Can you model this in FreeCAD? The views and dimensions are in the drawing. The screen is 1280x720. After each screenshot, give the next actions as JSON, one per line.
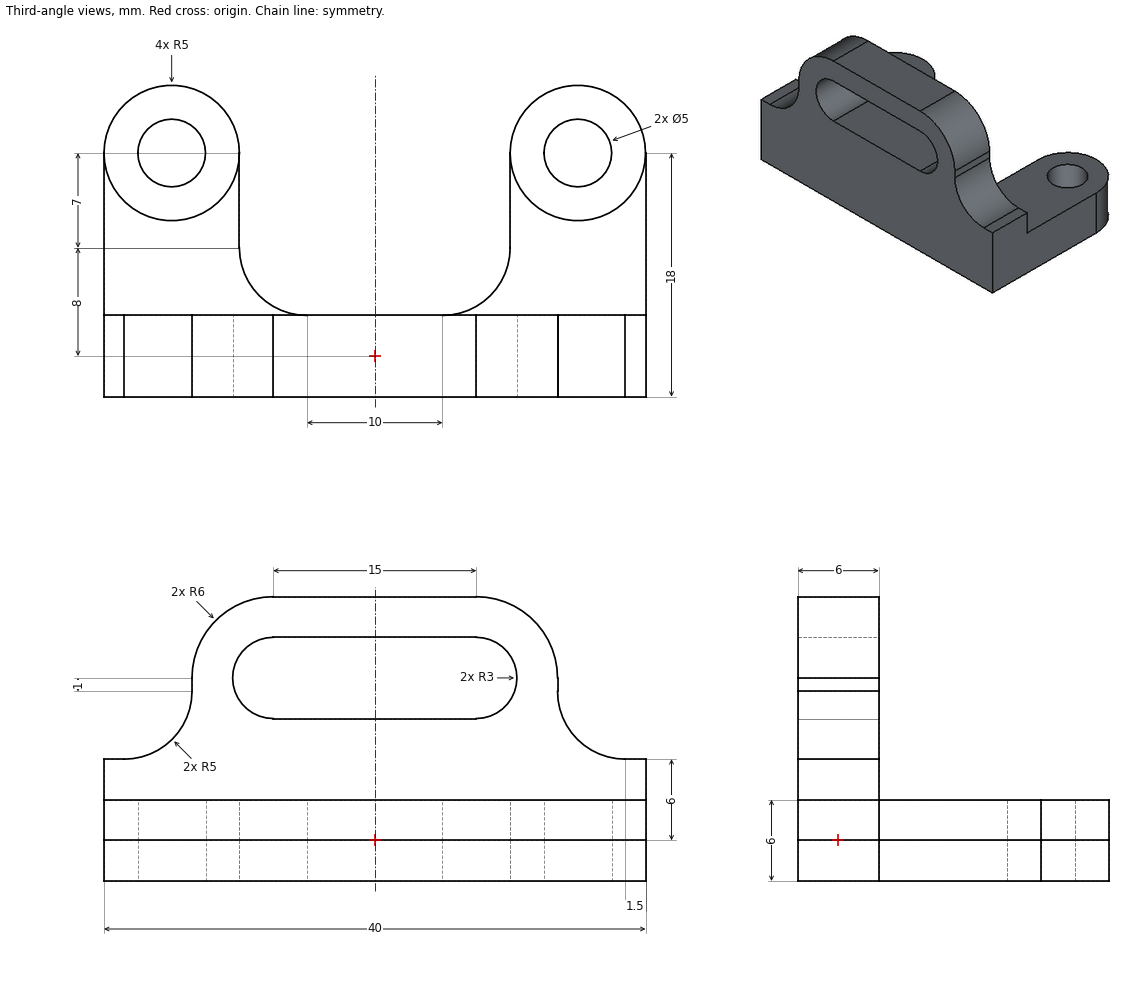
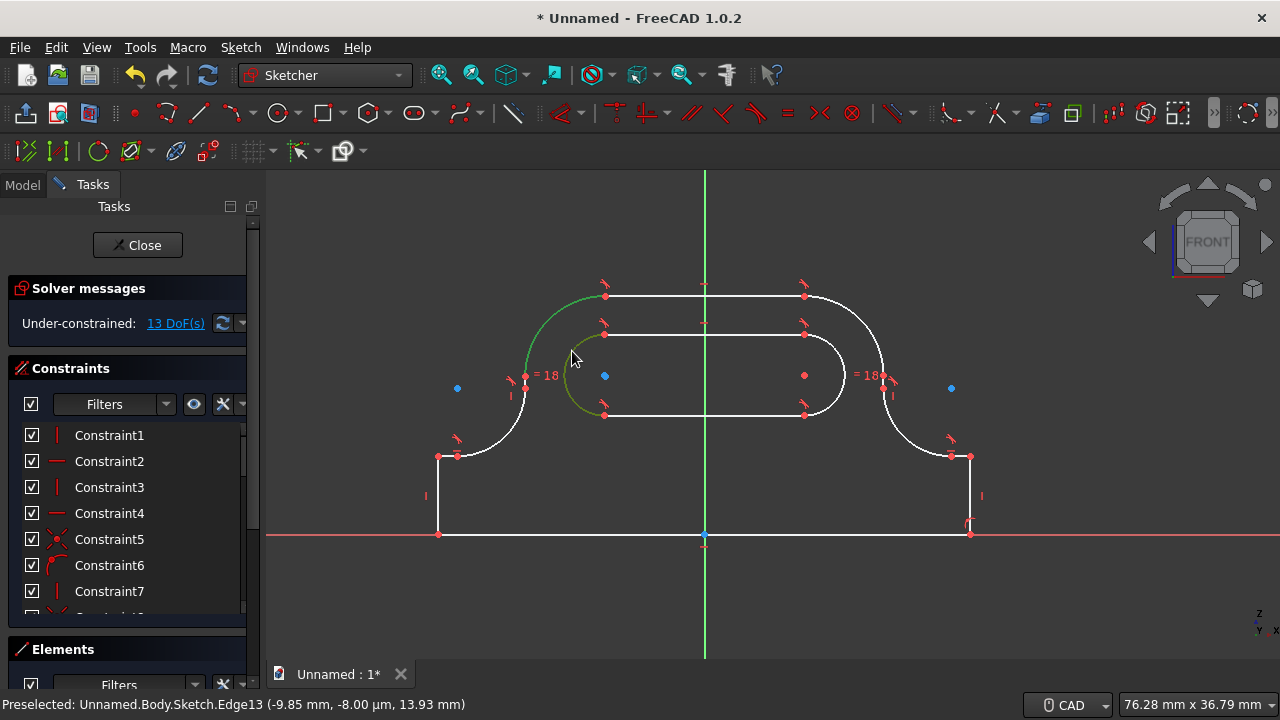
{"action": "left_click", "coordinate": [616, 114]}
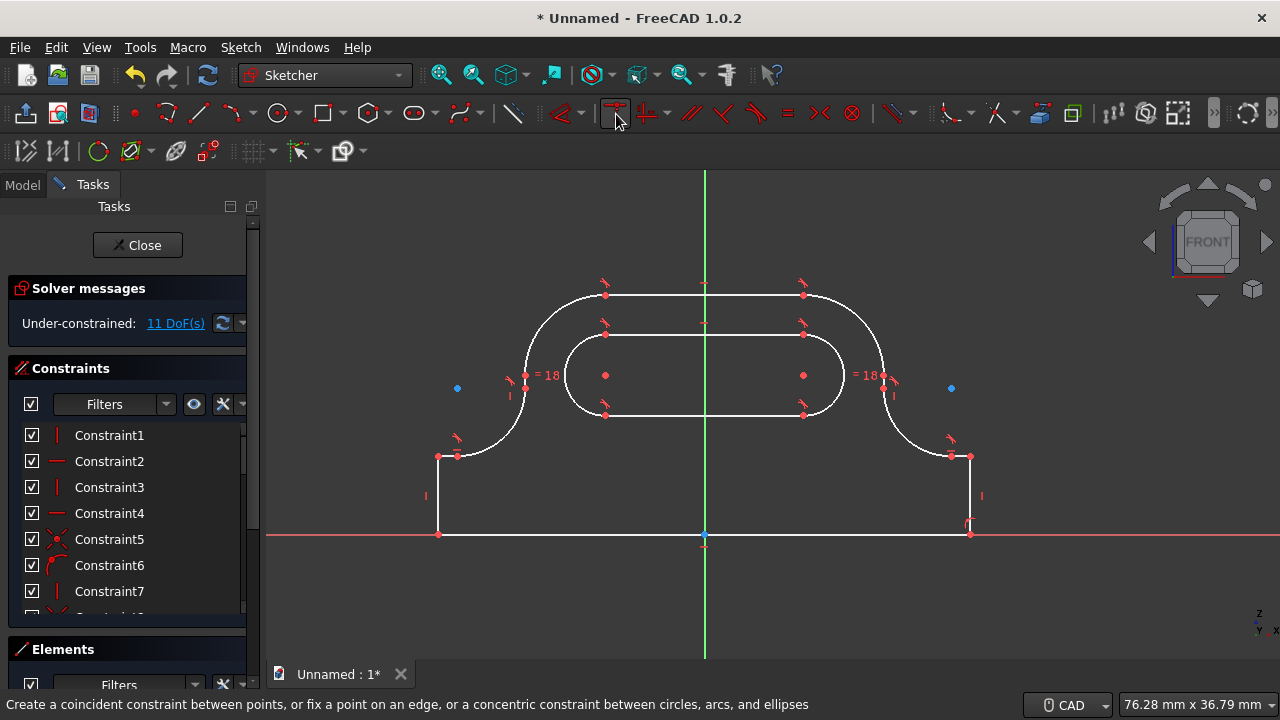
{"action": "left_click", "coordinate": [891, 419]}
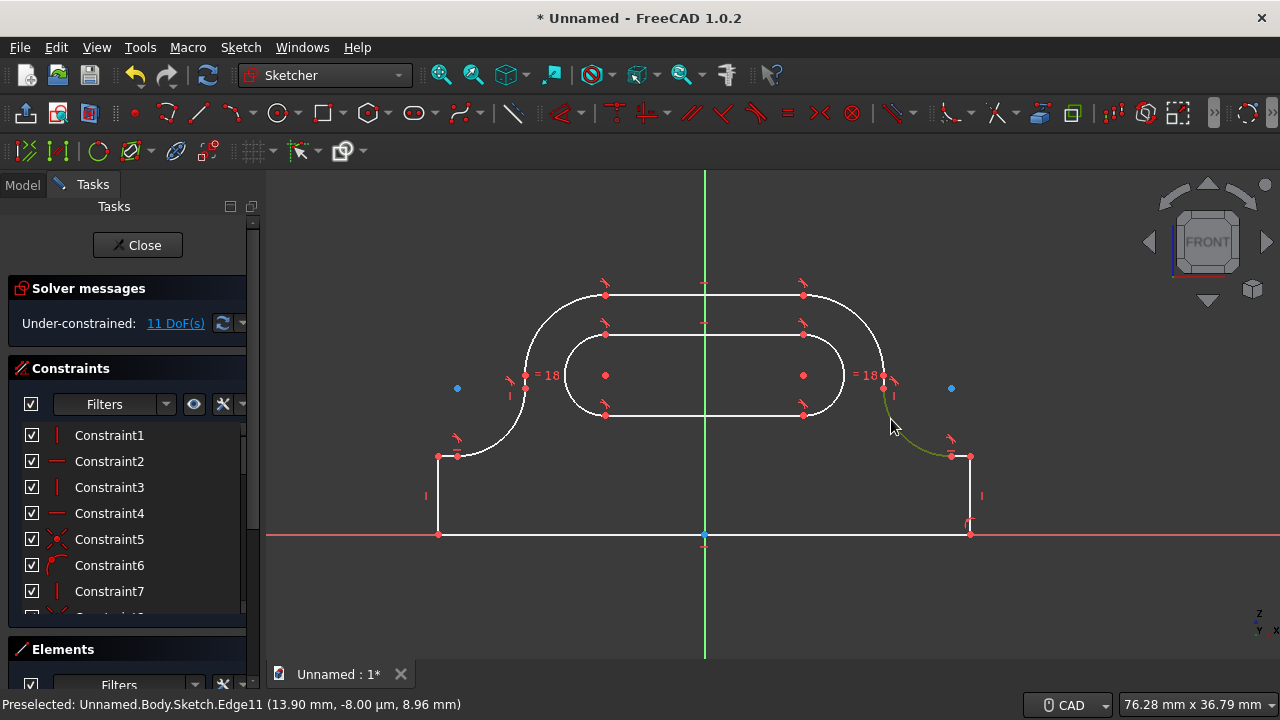
{"action": "left_click", "coordinate": [488, 449]}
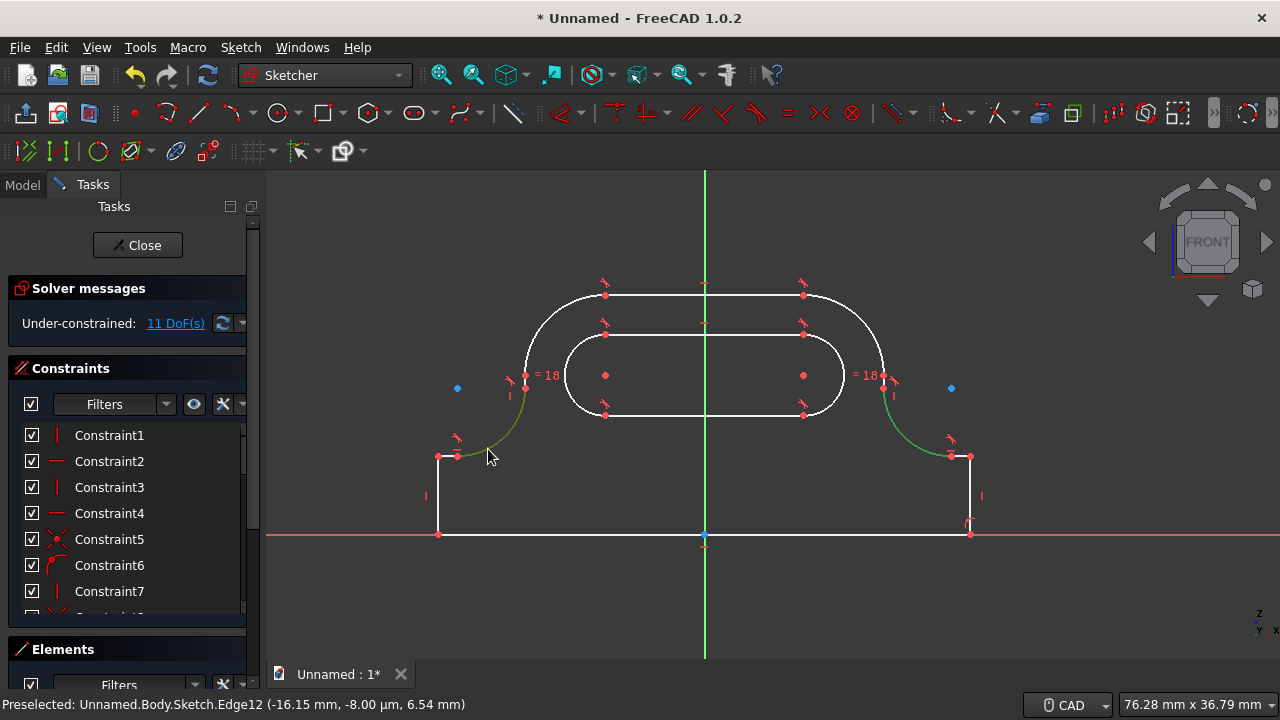
{"action": "left_click", "coordinate": [788, 114]}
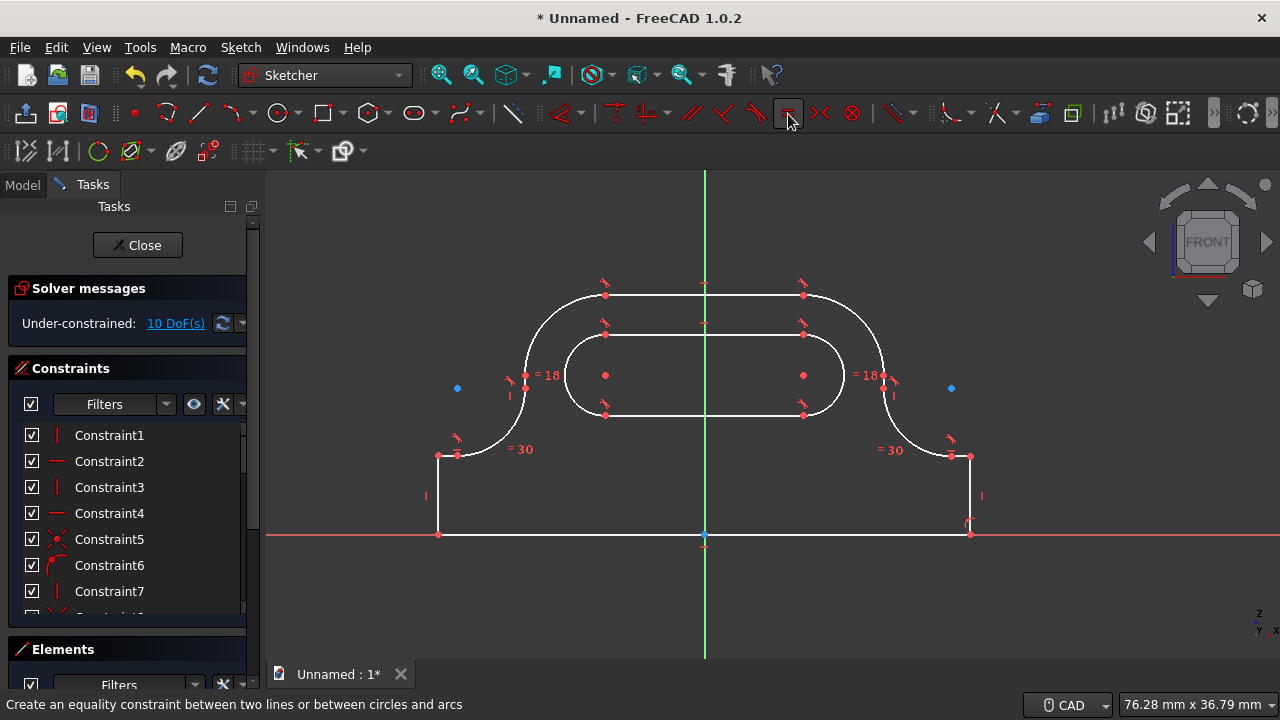
{"action": "left_click", "coordinate": [952, 388]}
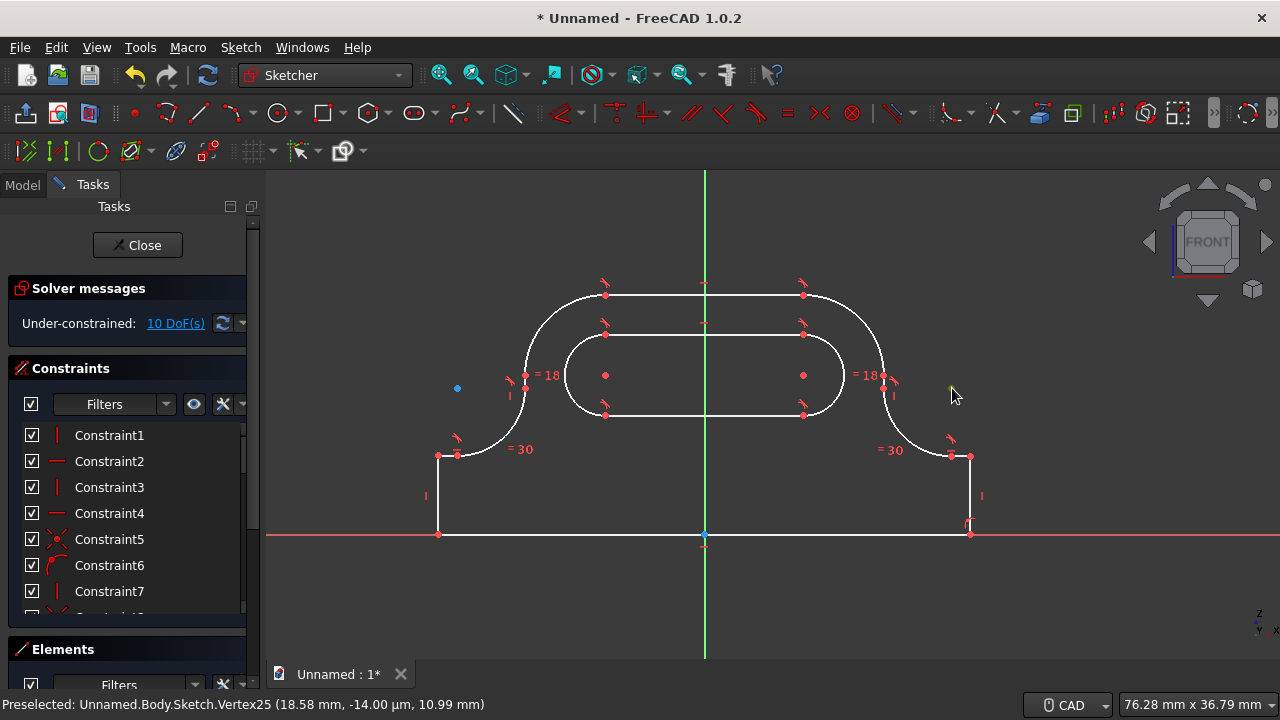
{"action": "left_click", "coordinate": [457, 388]}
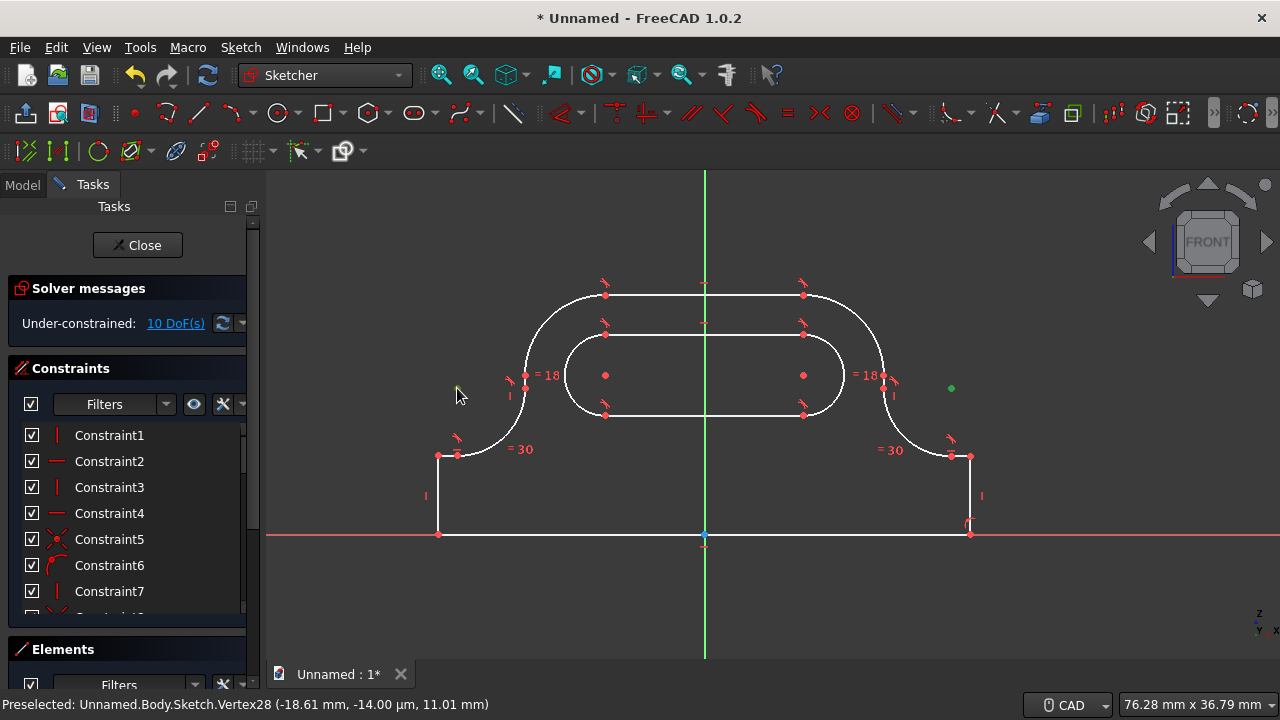
{"action": "left_click", "coordinate": [705, 600]}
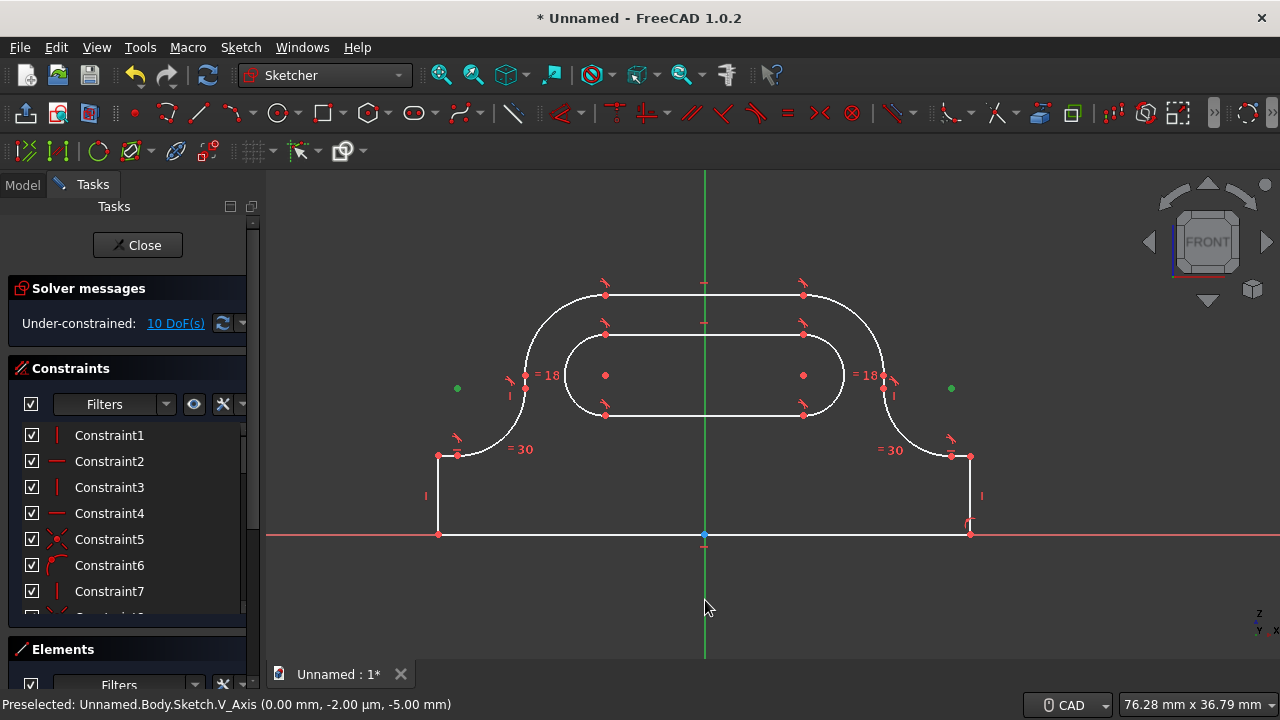
{"action": "key", "text": "s"}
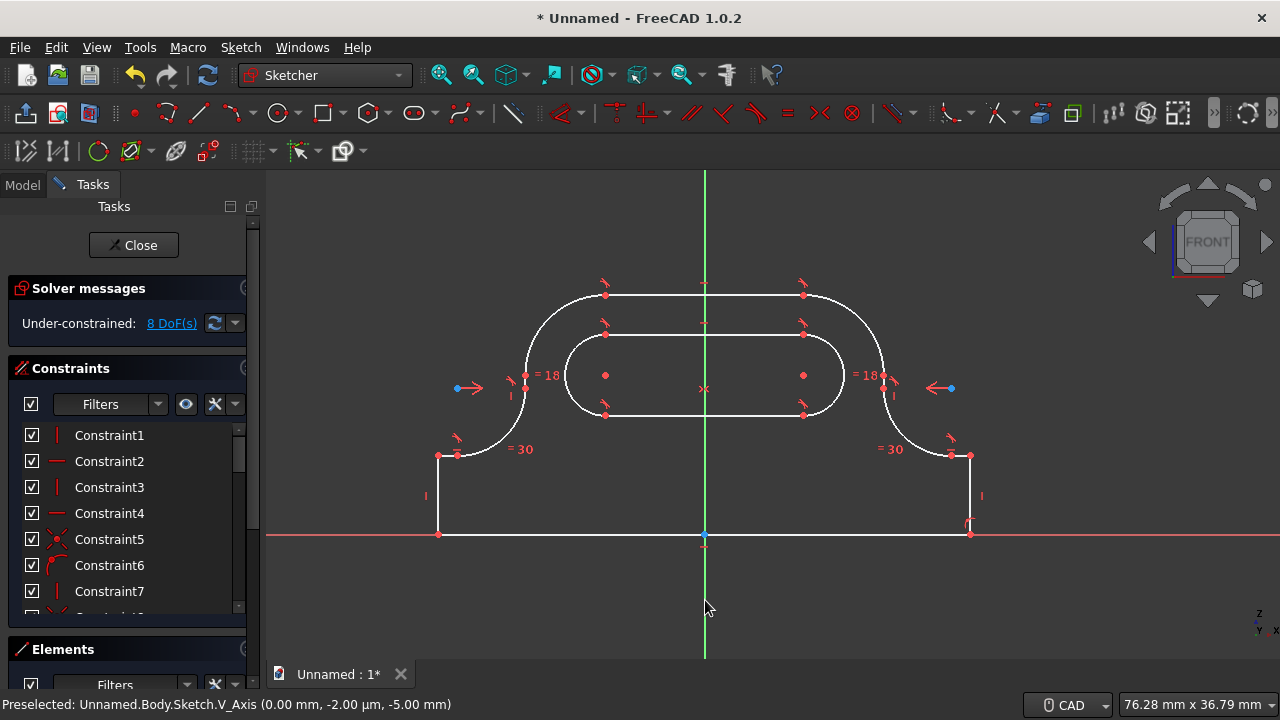
{"action": "left_click", "coordinate": [560, 114]}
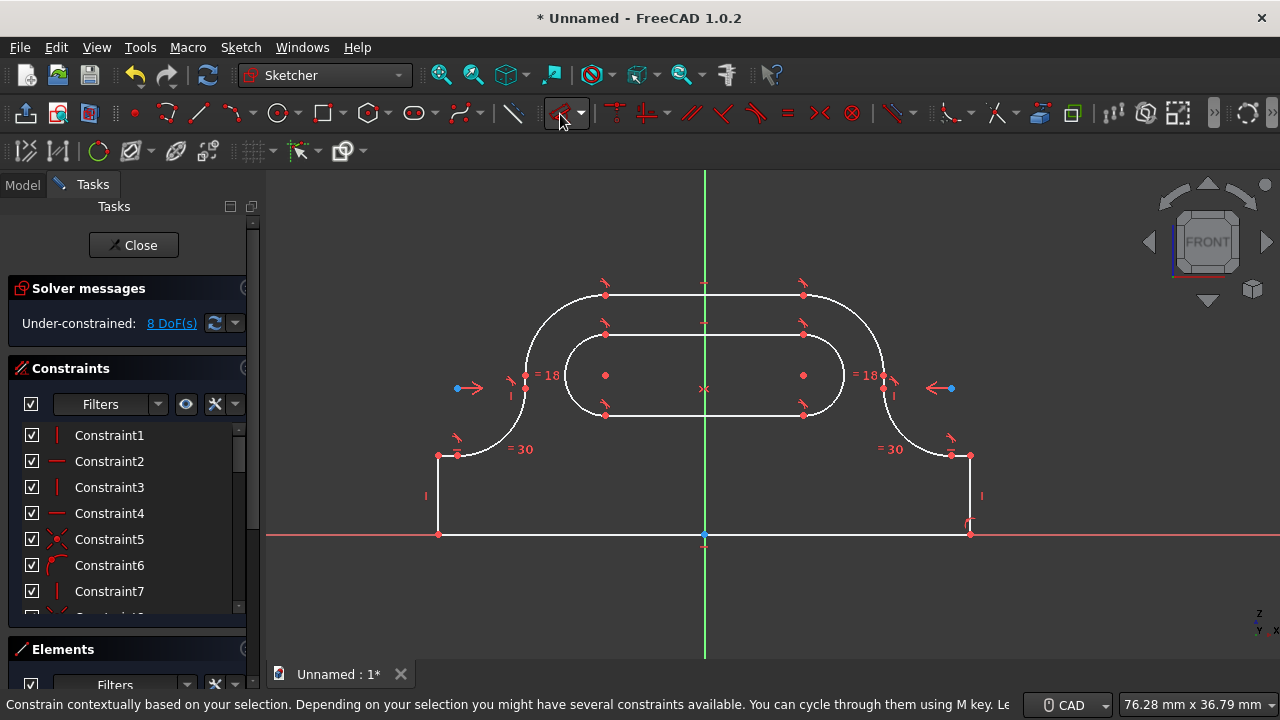
{"action": "left_click", "coordinate": [569, 304]}
{"action": "left_click", "coordinate": [554, 276]}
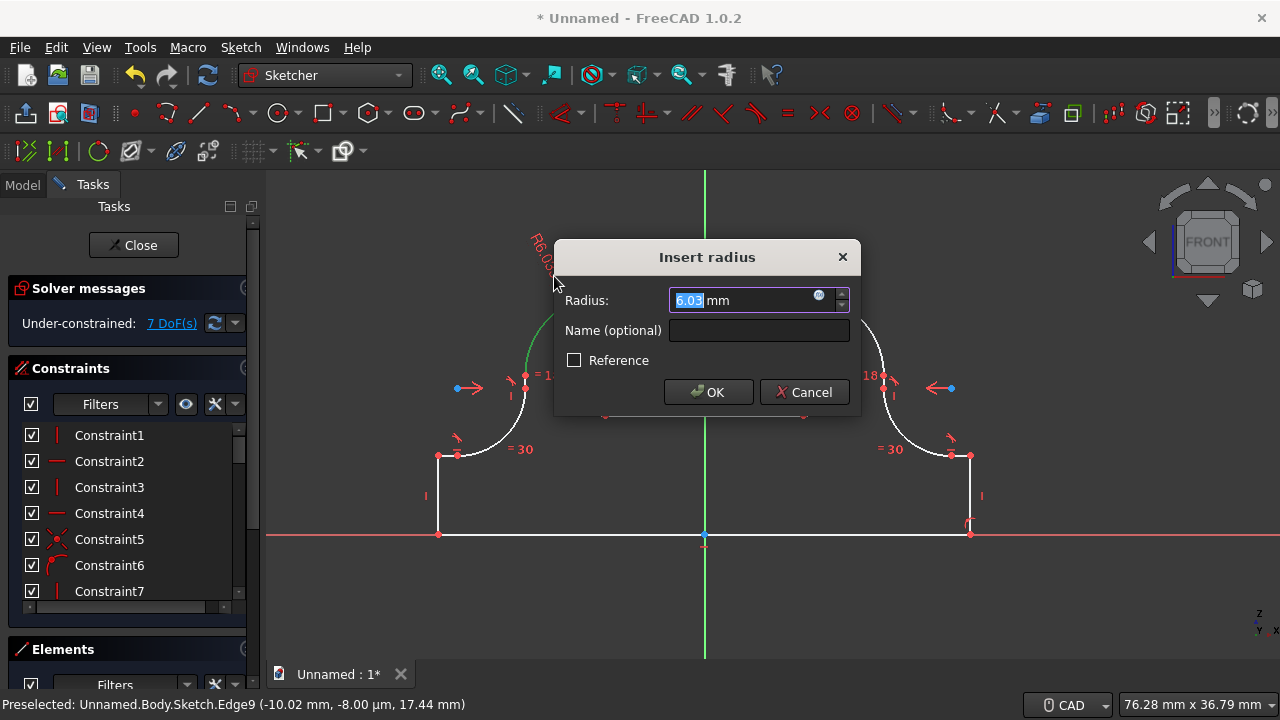
{"action": "type", "text": "6"}
{"action": "key", "text": "Return"}